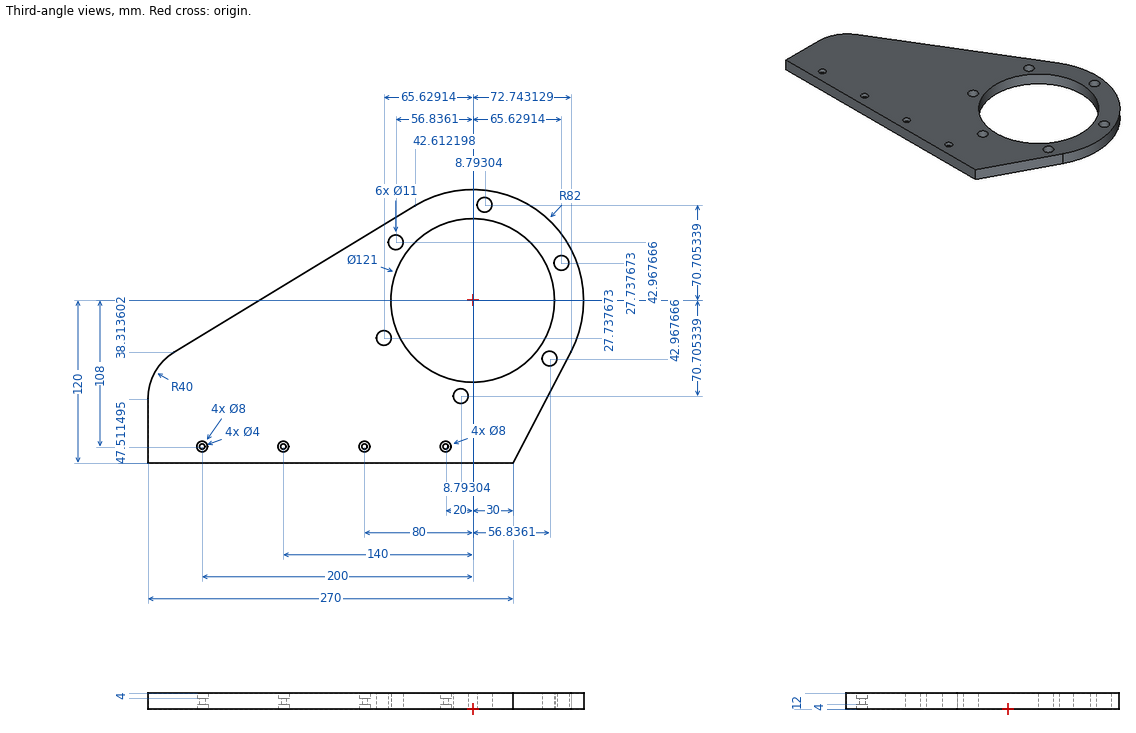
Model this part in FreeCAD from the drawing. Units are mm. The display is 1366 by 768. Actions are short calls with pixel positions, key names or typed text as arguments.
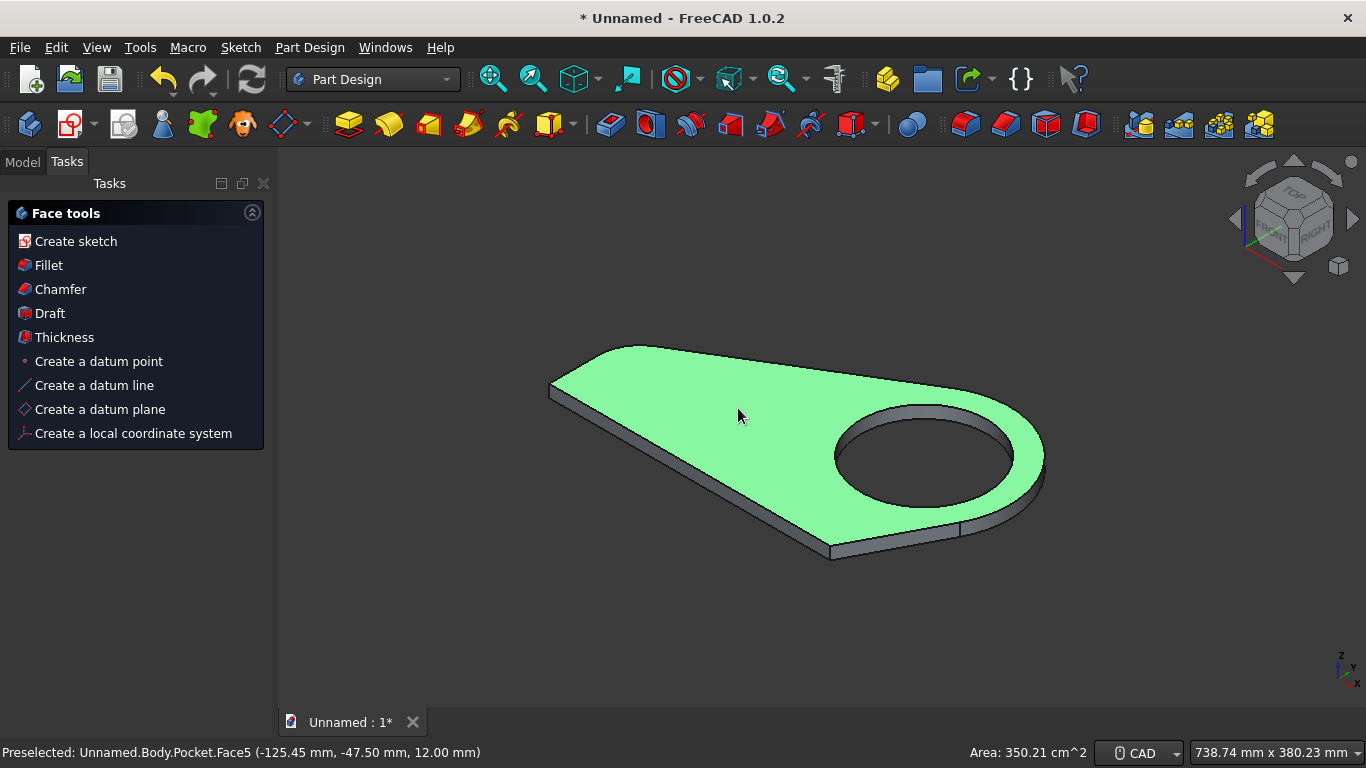
click(70, 124)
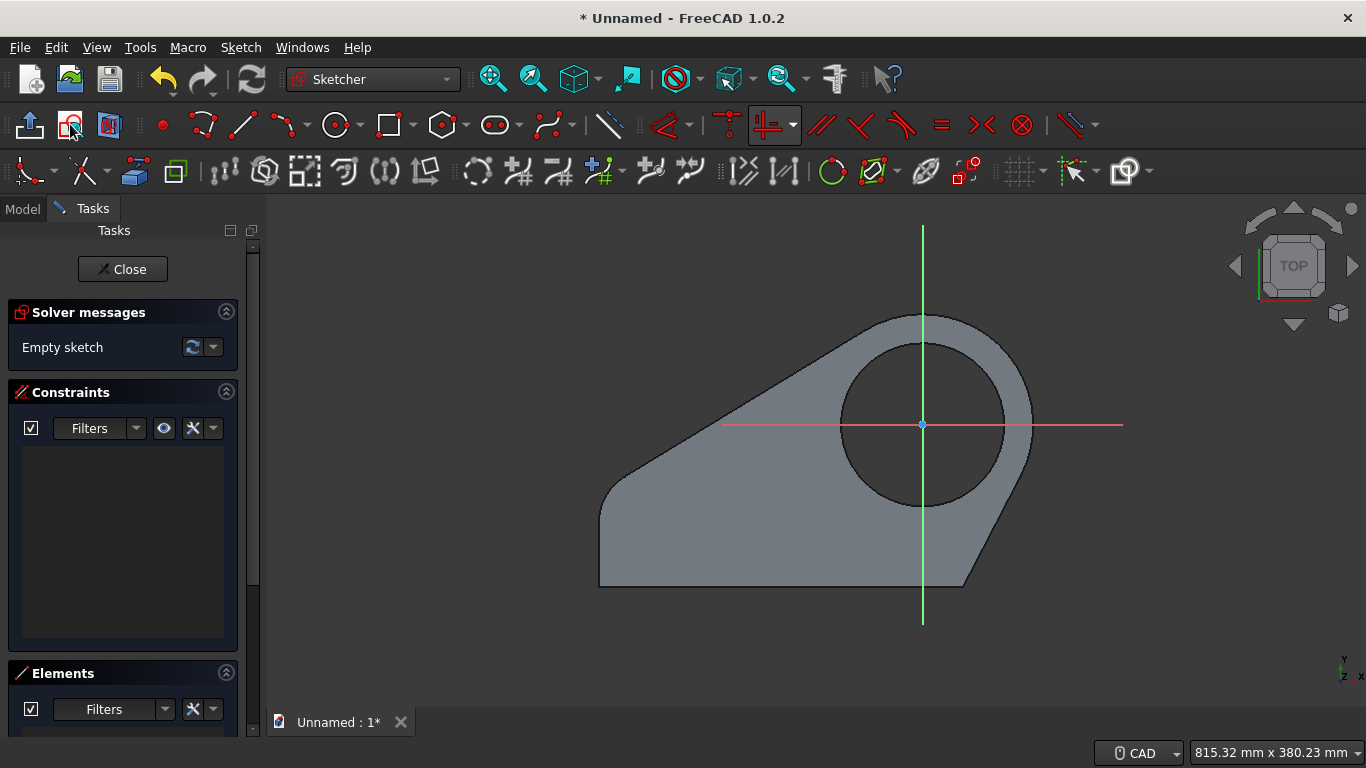
scroll(818, 539, up, 4)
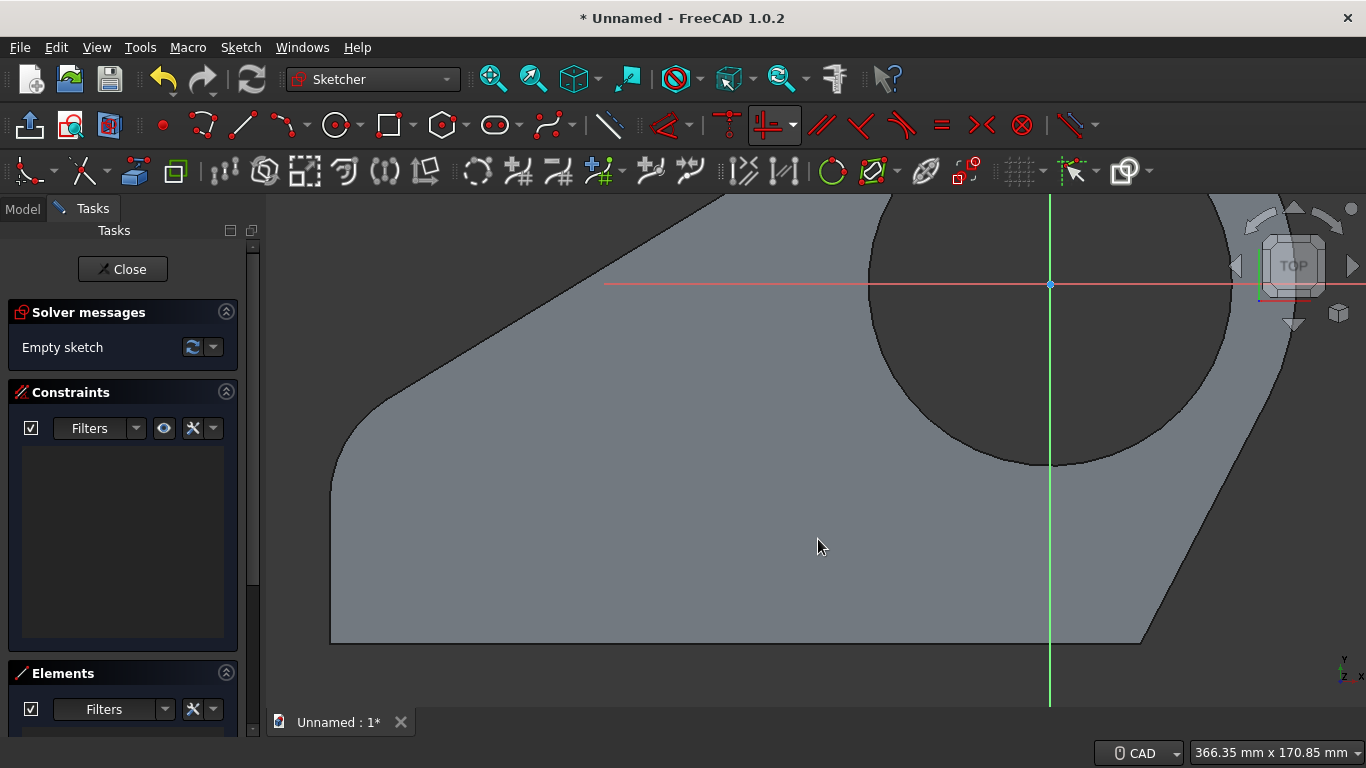
click(336, 126)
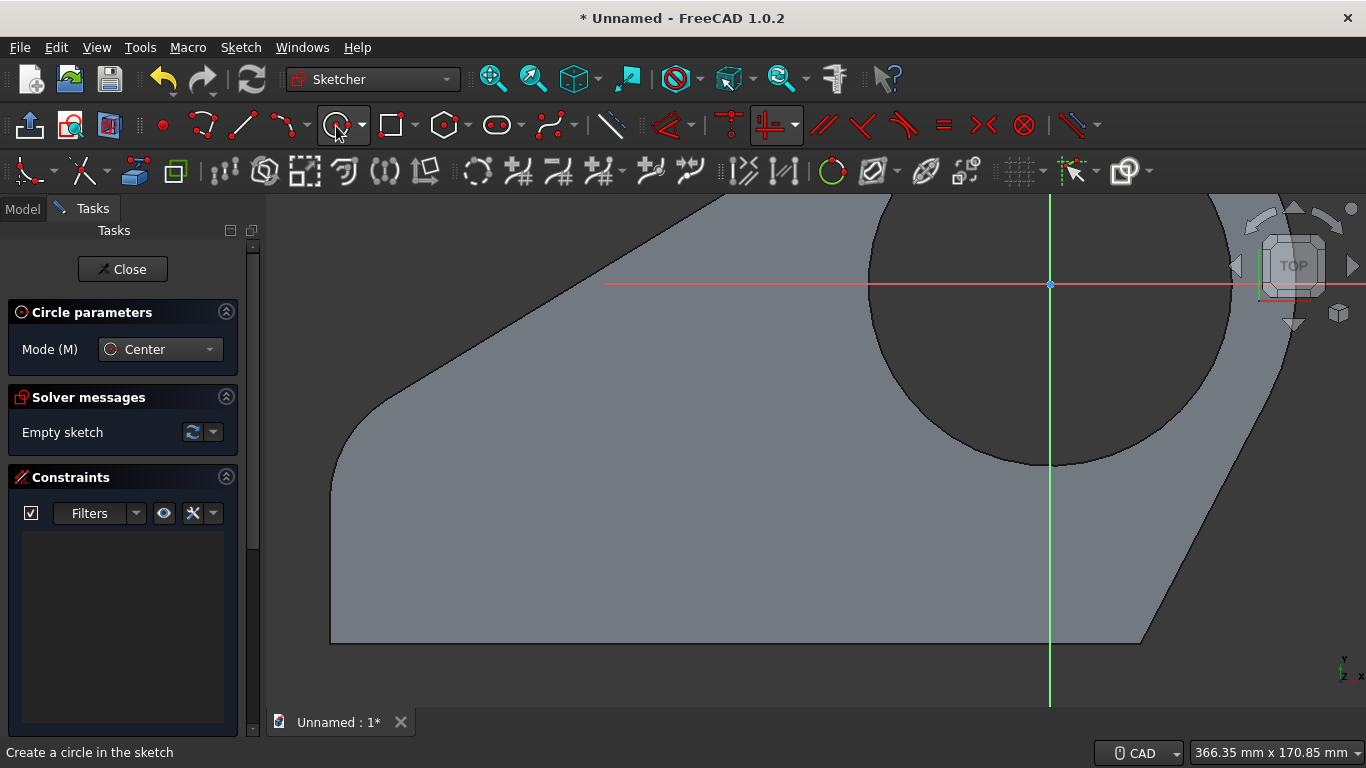
scroll(450, 608, up, 7)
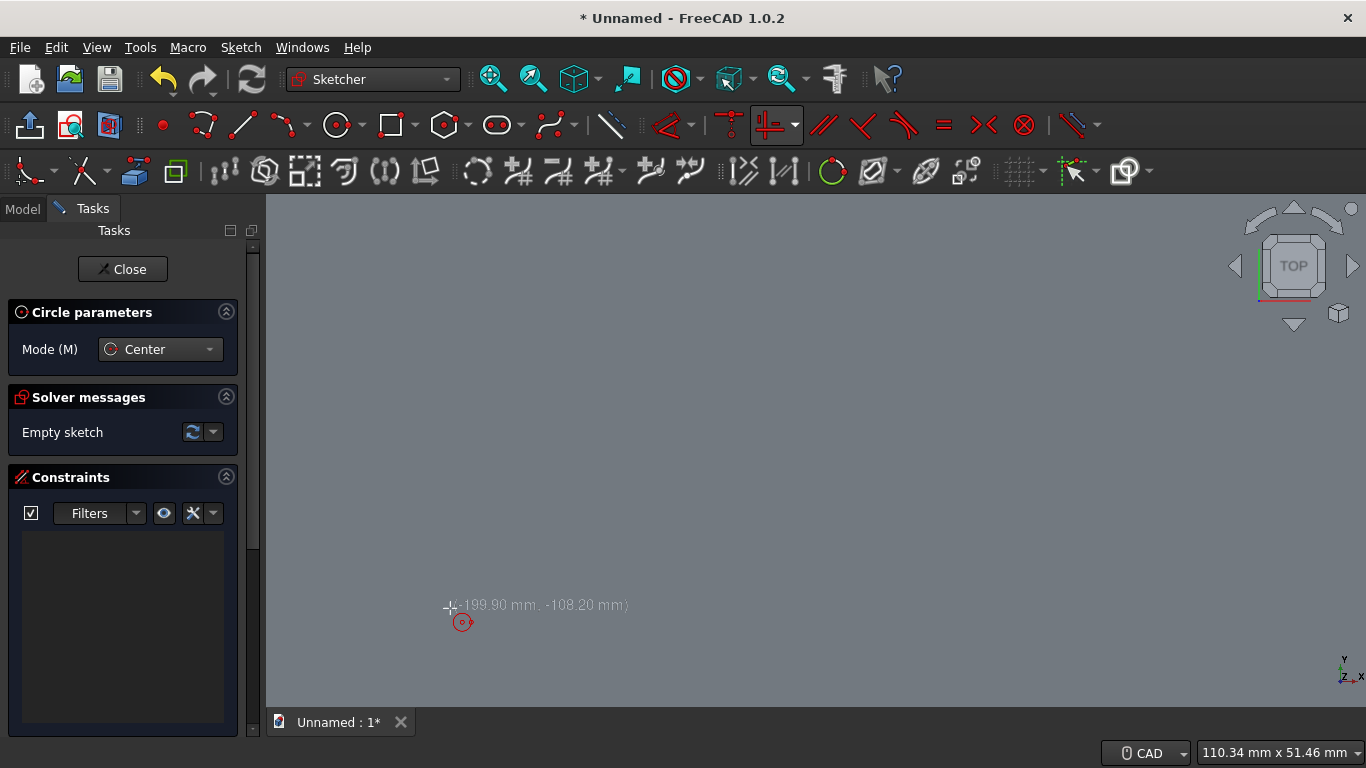
scroll(451, 610, down, 7)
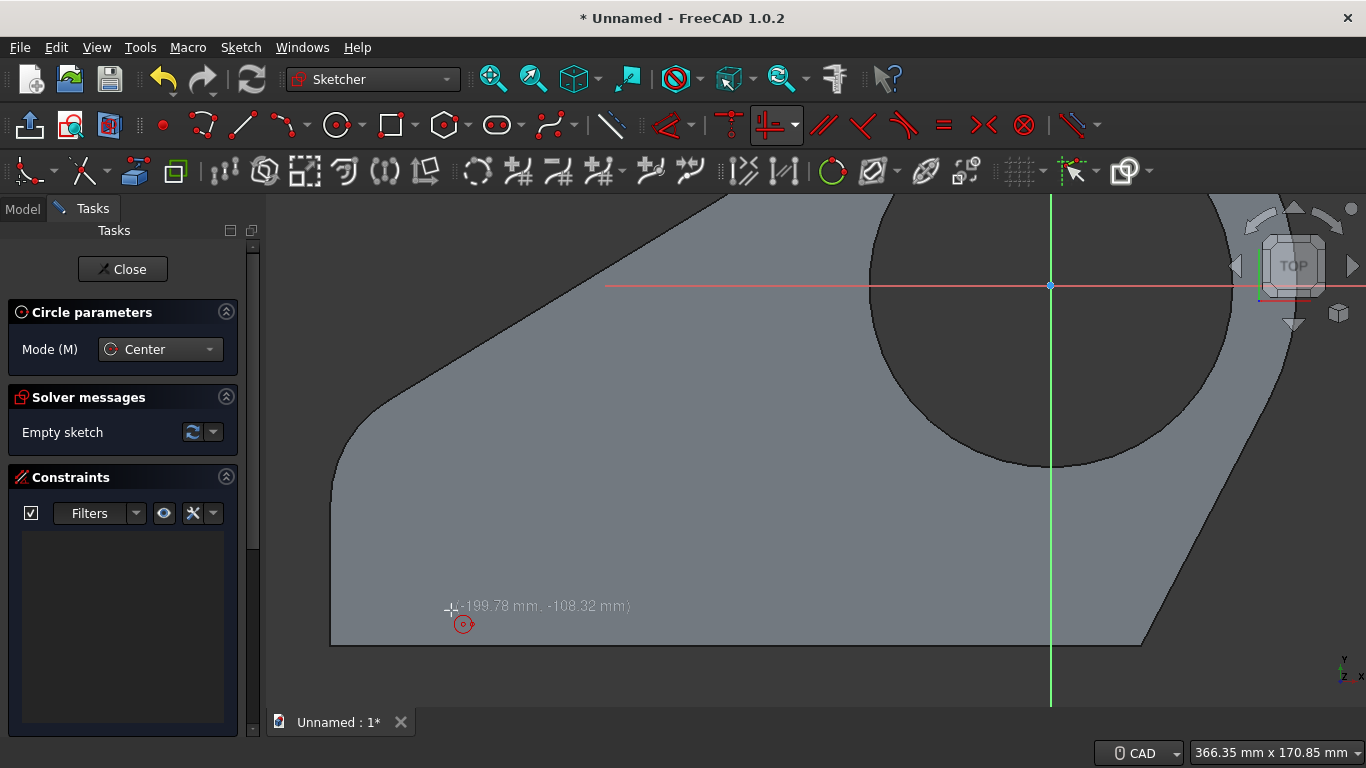
click(450, 610)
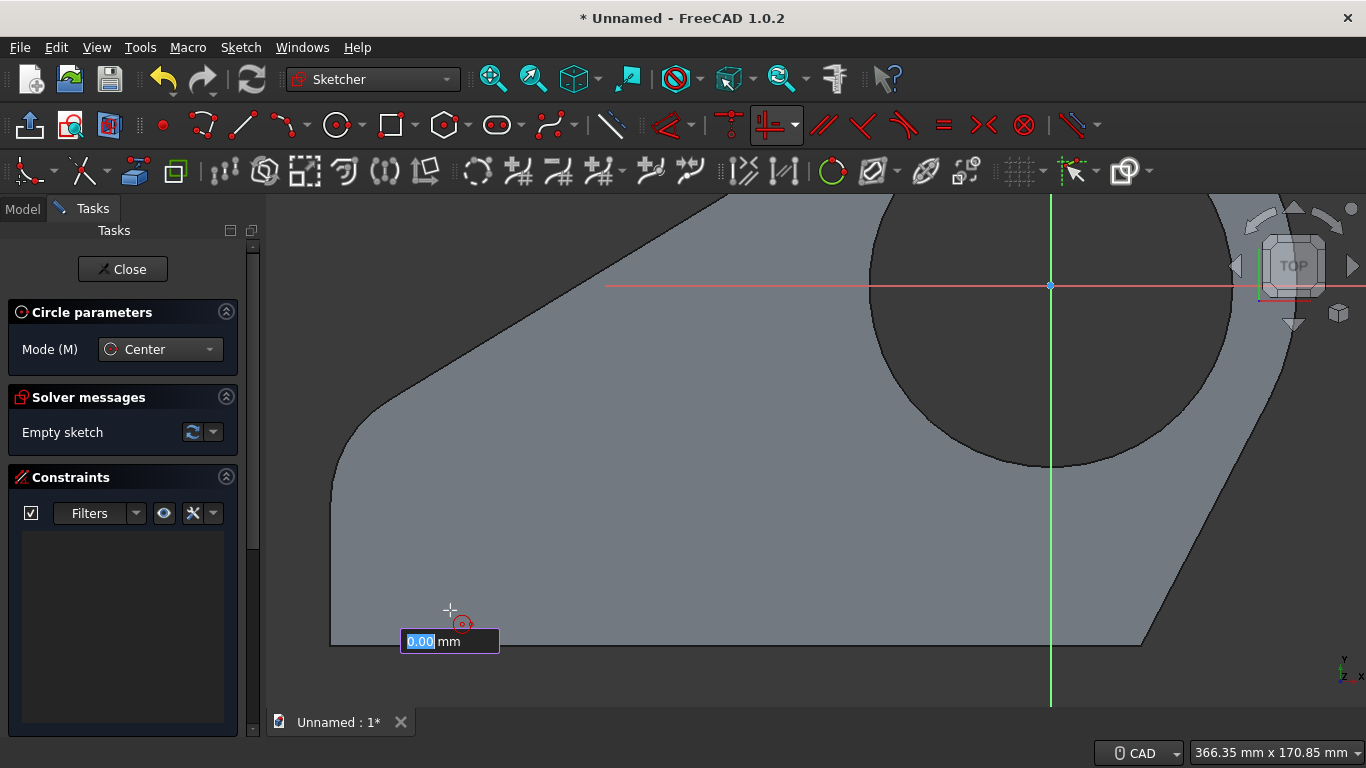
scroll(455, 606, up, 5)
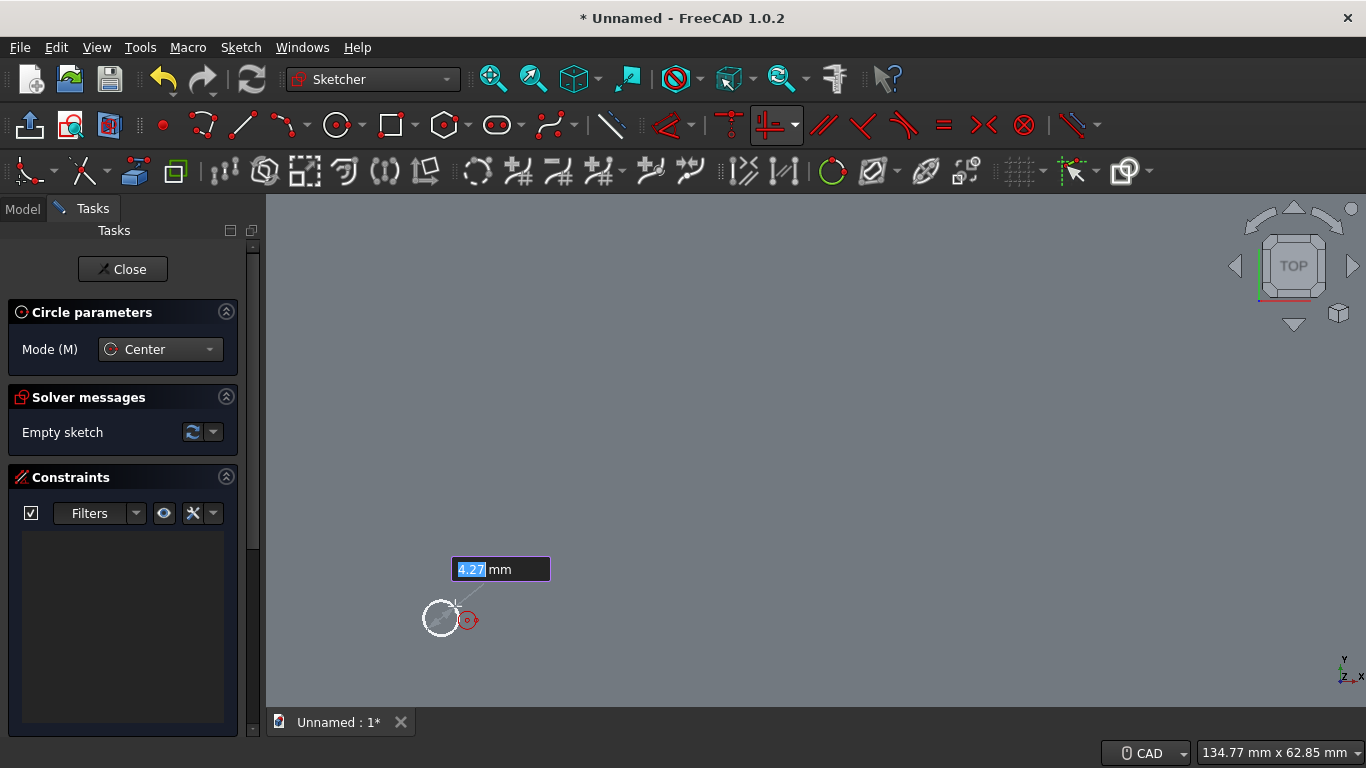
click(454, 604)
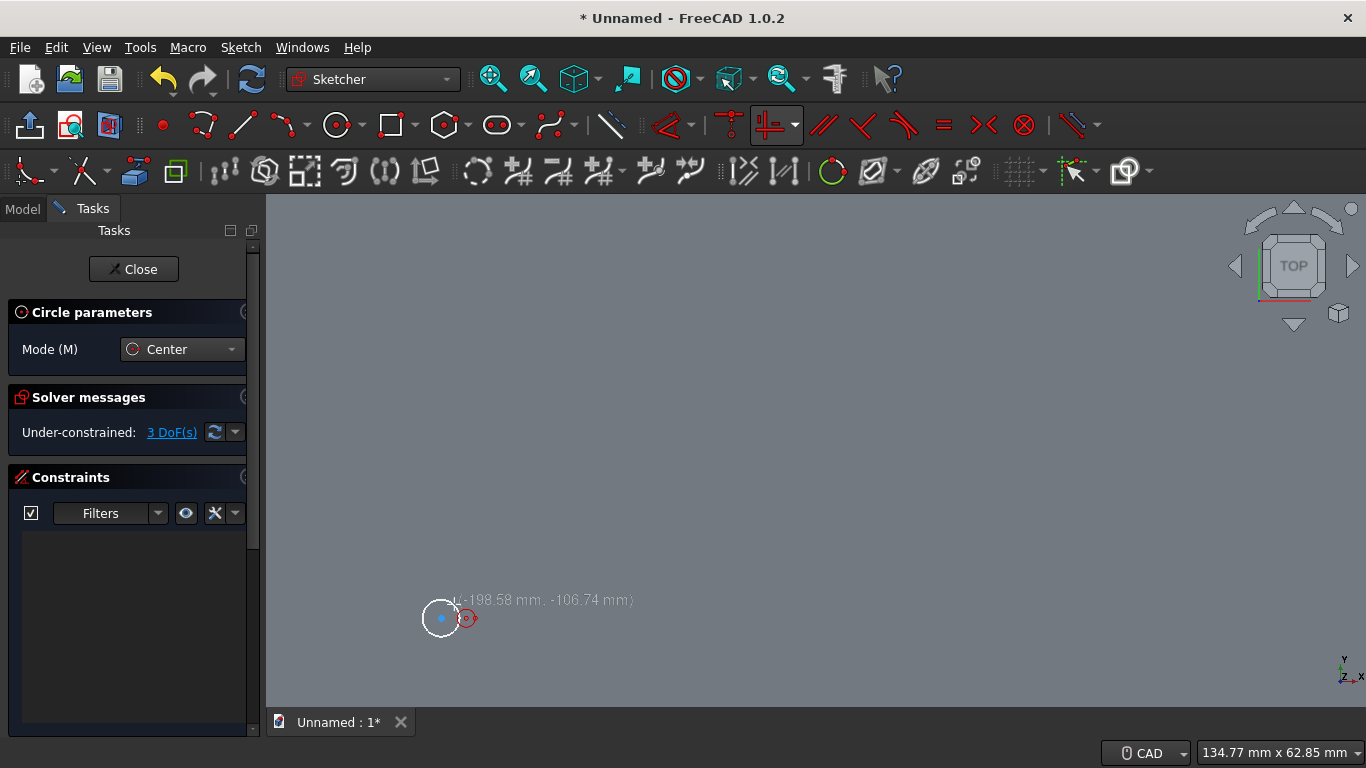
scroll(932, 615, up, 2)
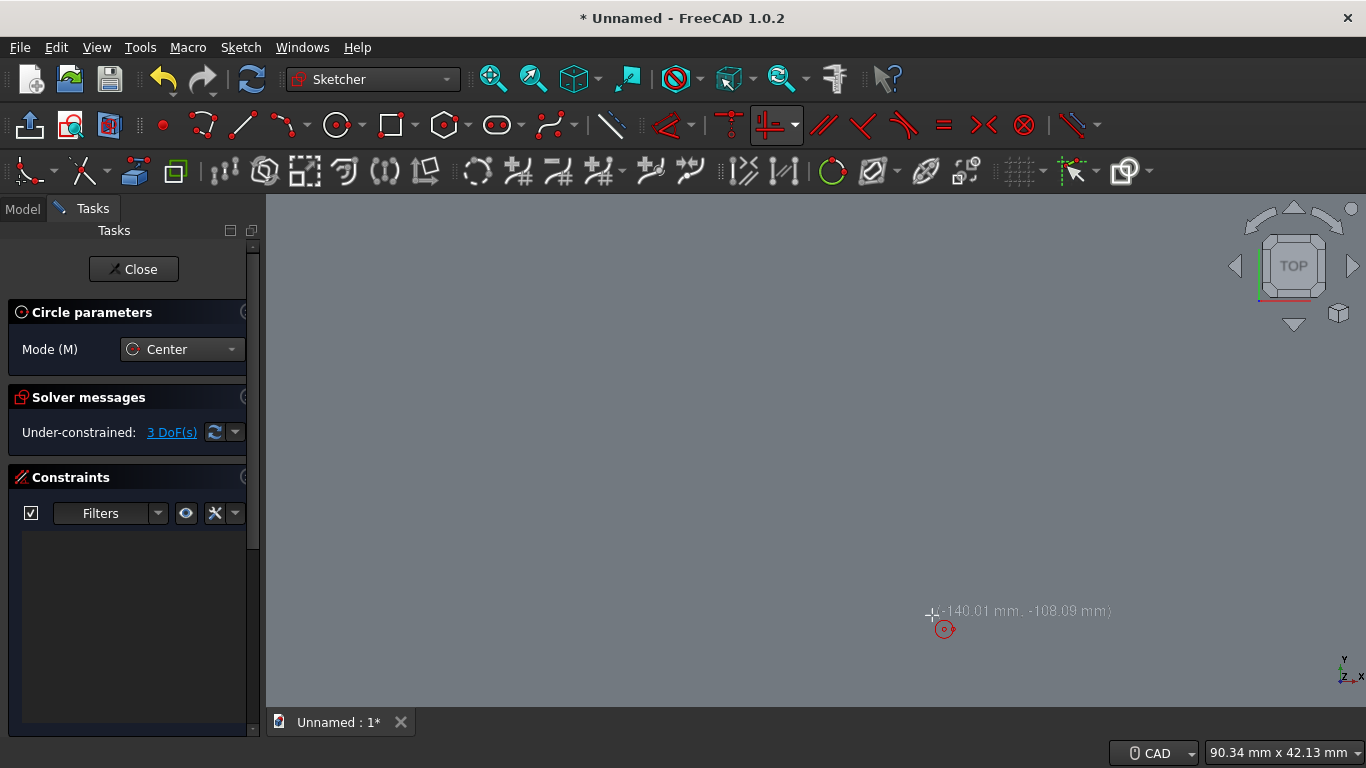
scroll(532, 608, down, 7)